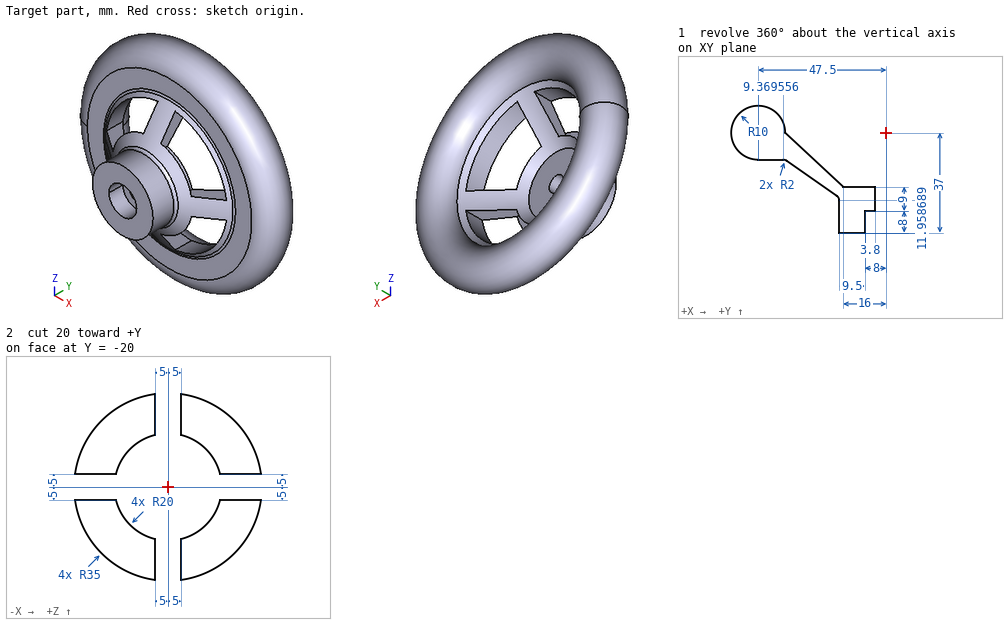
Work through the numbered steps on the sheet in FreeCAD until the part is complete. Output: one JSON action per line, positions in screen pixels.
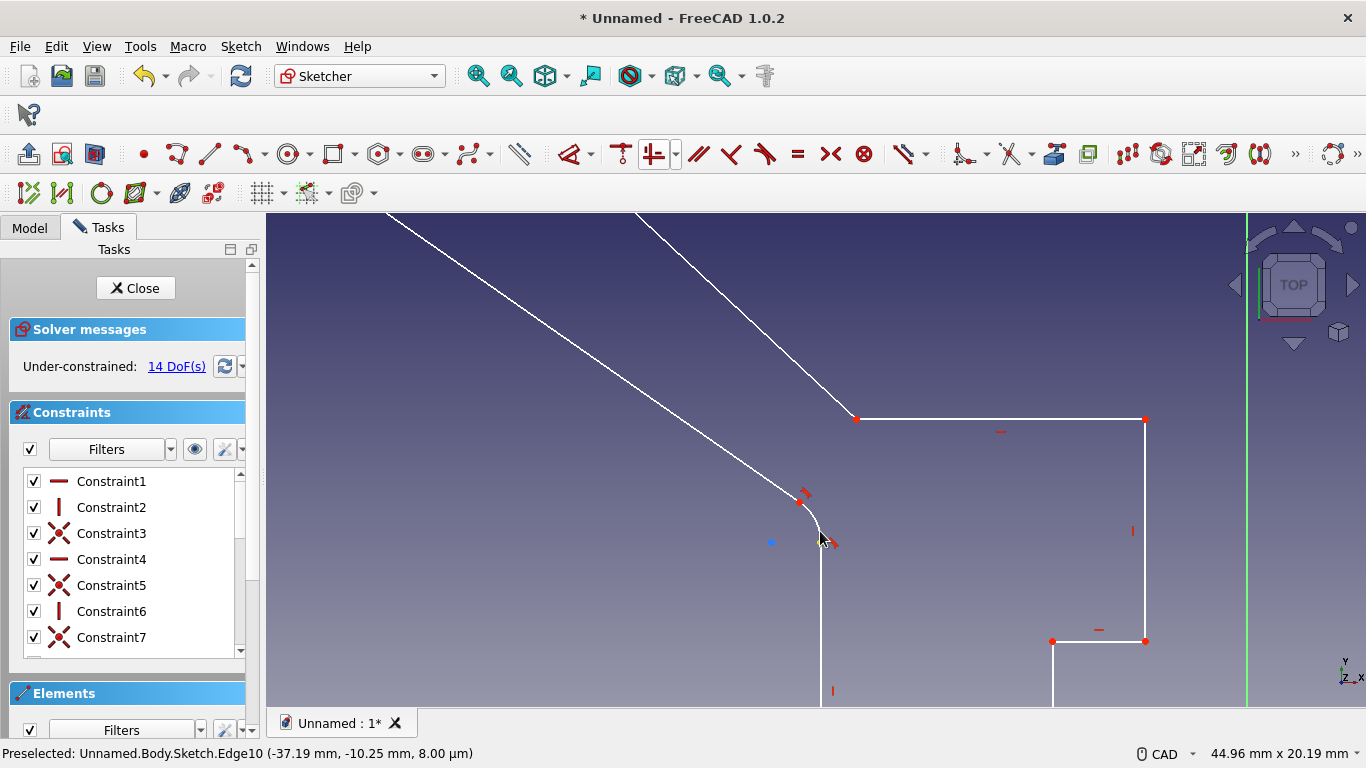
{"action": "left_click", "coordinate": [819, 529]}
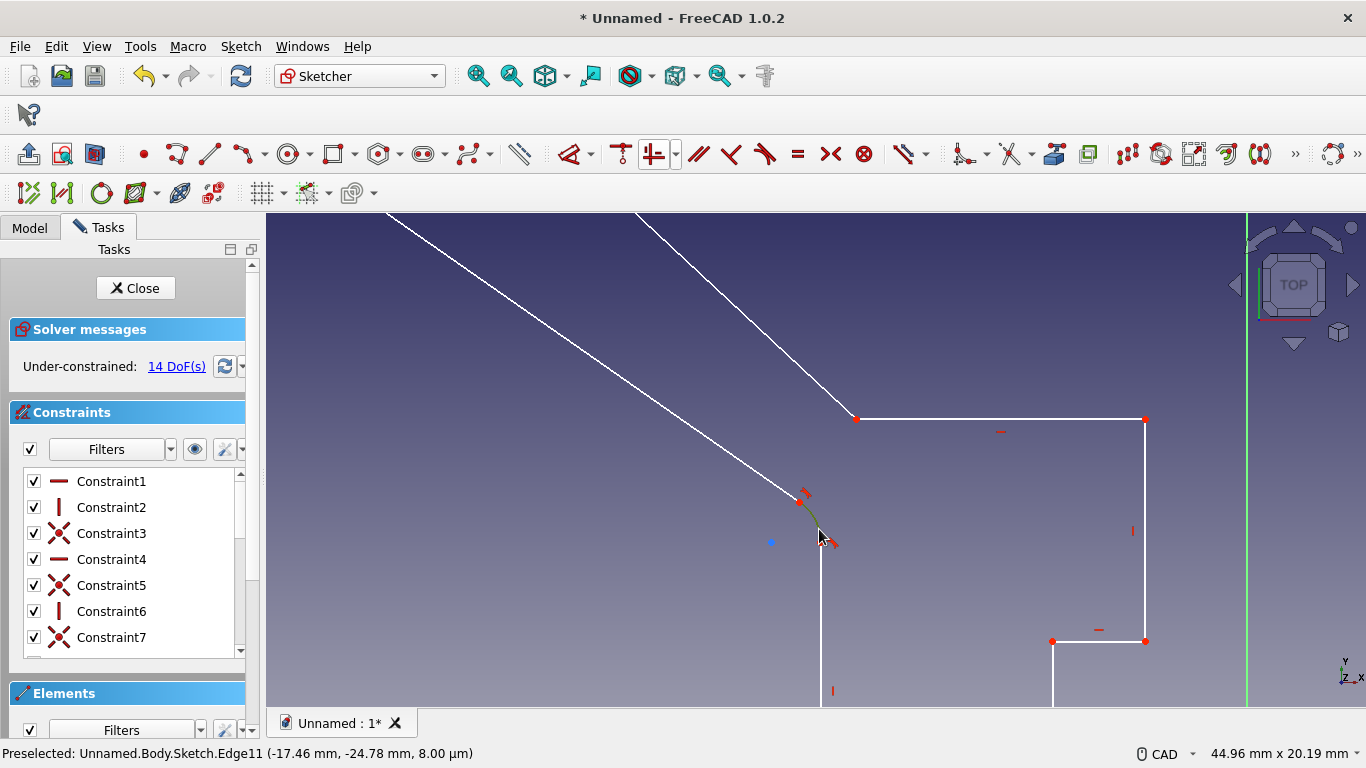
{"action": "key", "text": "e"}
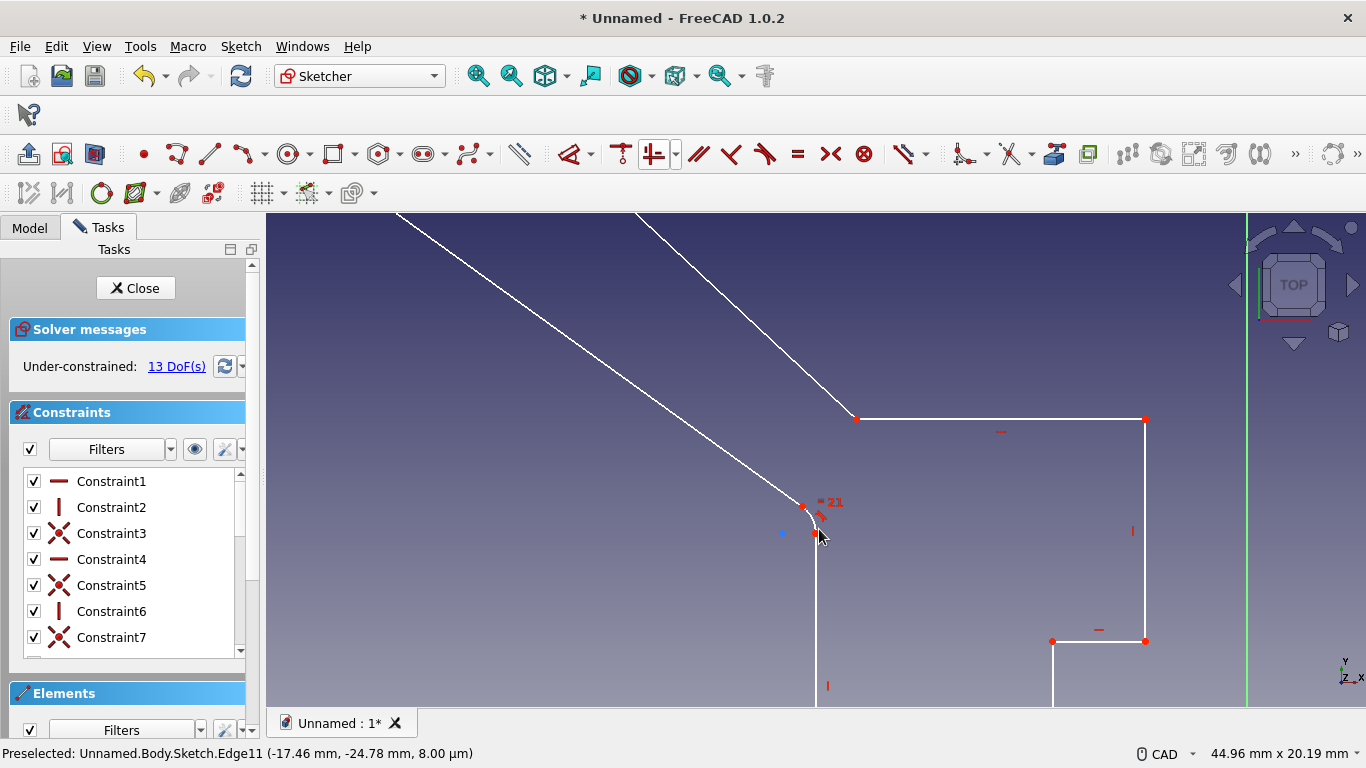
{"action": "scroll", "coordinate": [820, 531], "scroll_direction": "down", "scroll_amount": 6}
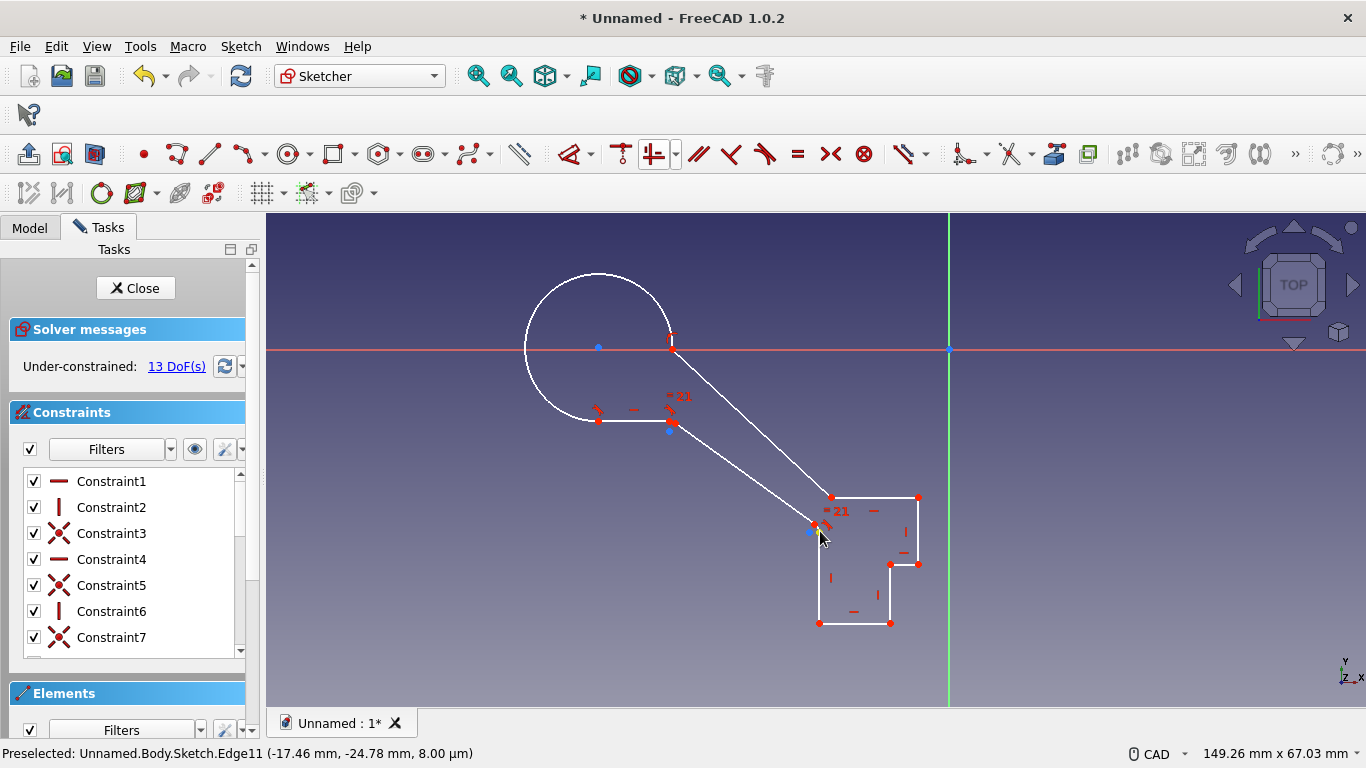
{"action": "left_click", "coordinate": [599, 348]}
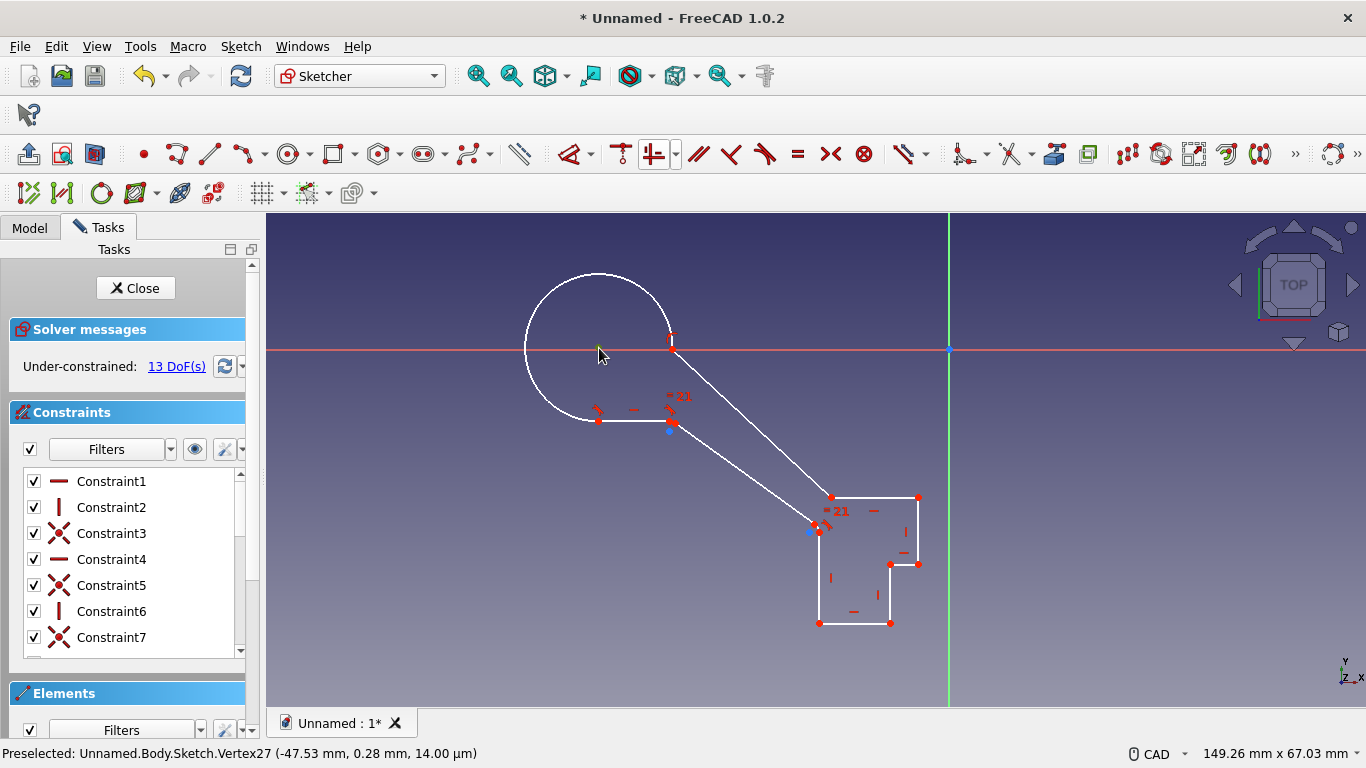
{"action": "left_click", "coordinate": [359, 350]}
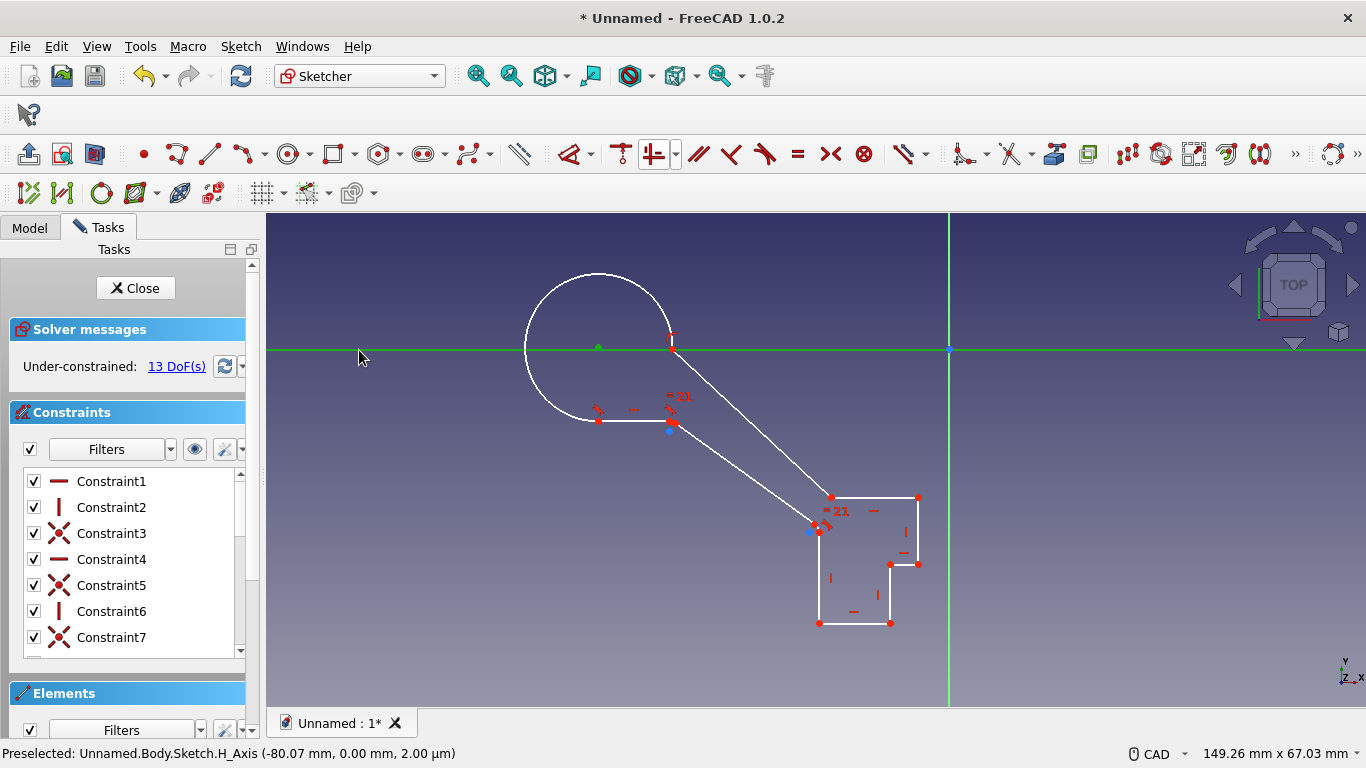
{"action": "key", "text": "c"}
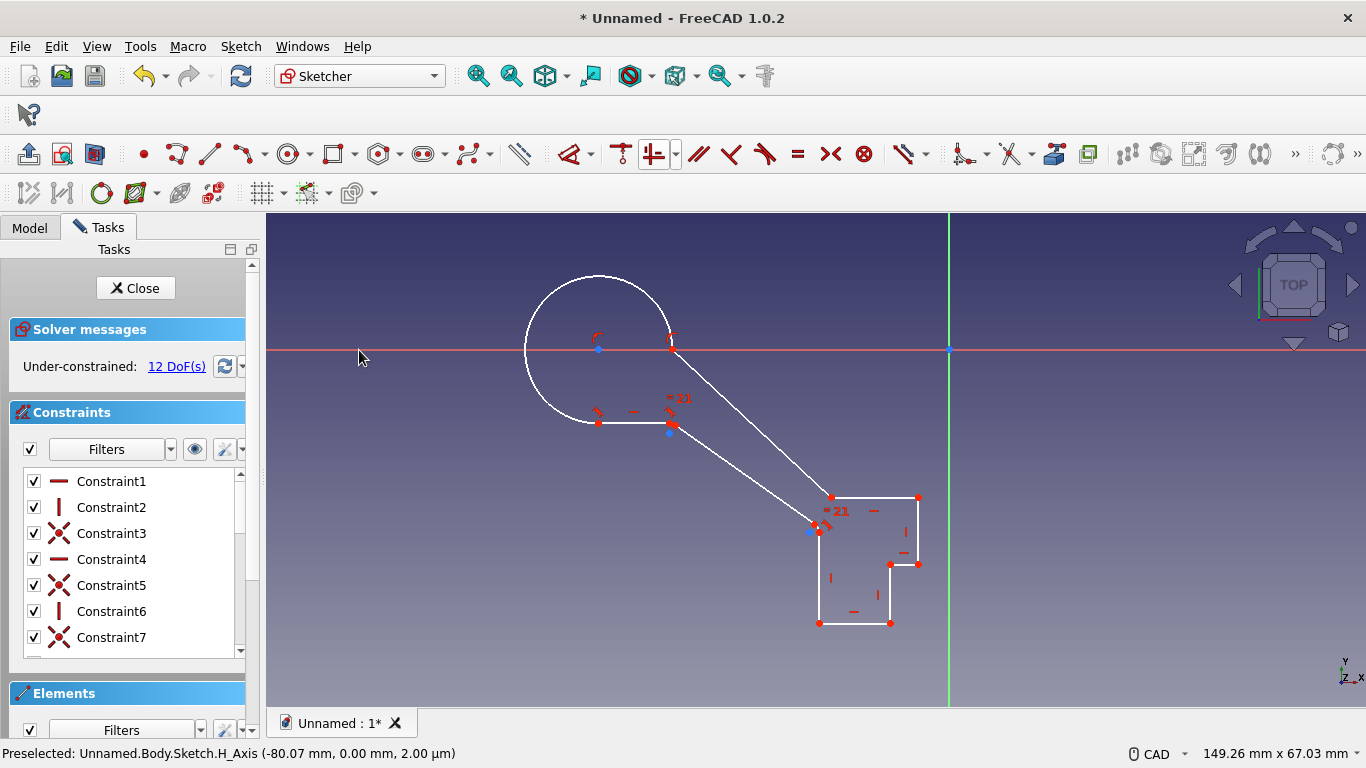
{"action": "key", "text": "d"}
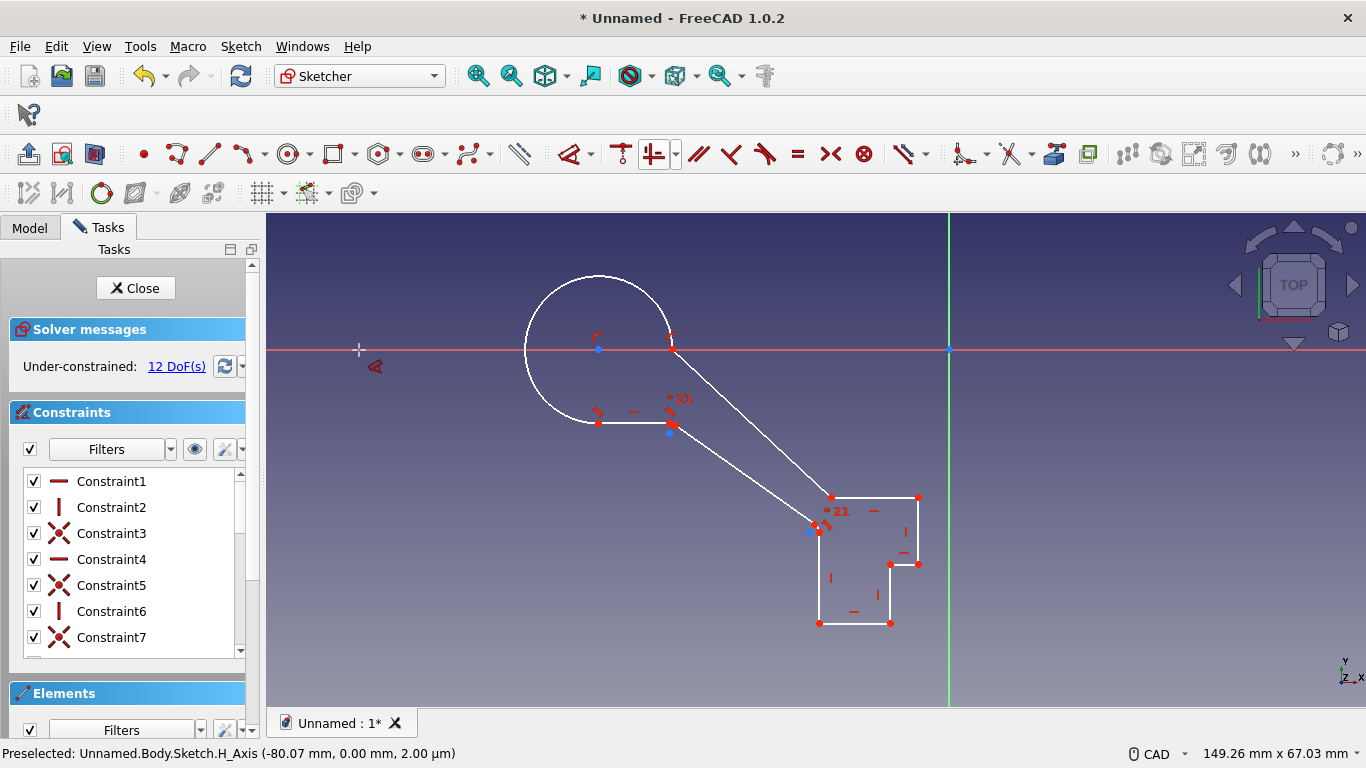
{"action": "scroll", "coordinate": [673, 424], "scroll_direction": "up", "scroll_amount": 8}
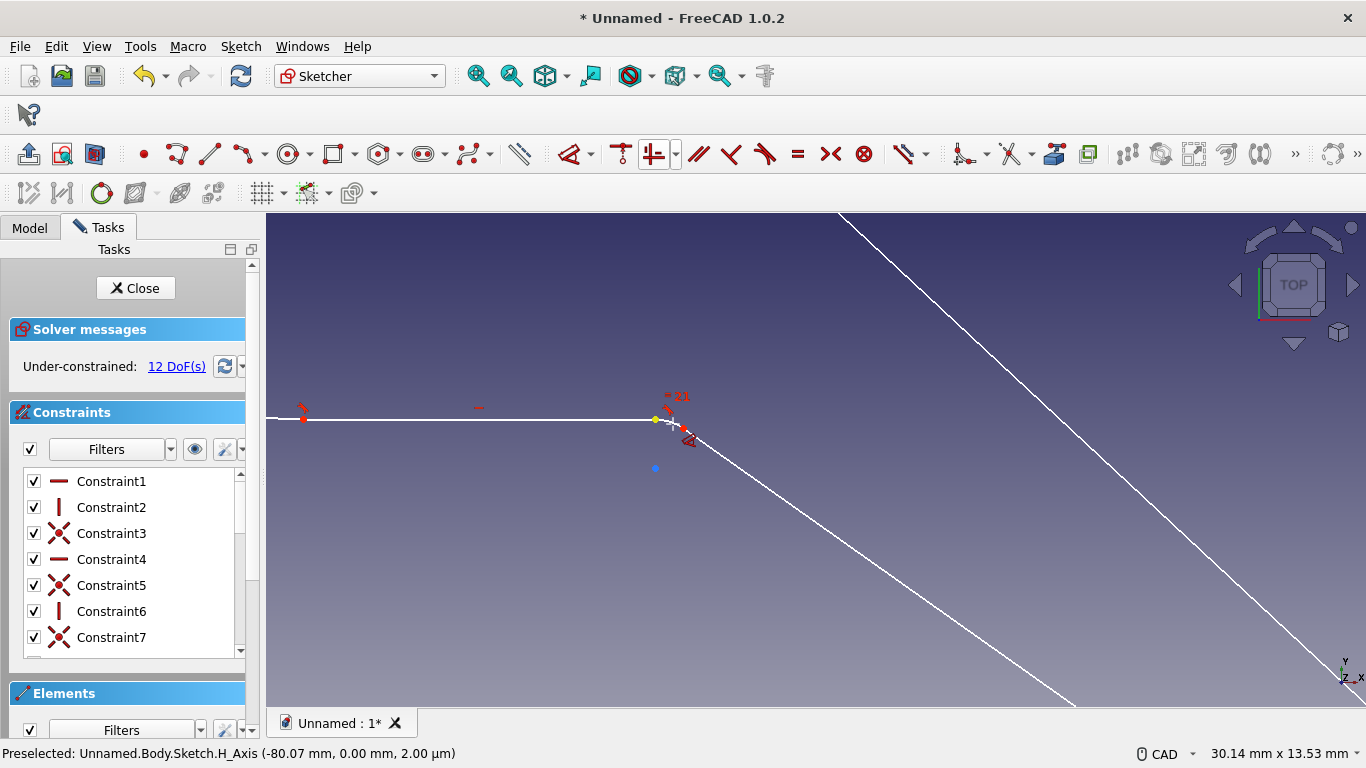
{"action": "left_click", "coordinate": [670, 422]}
{"action": "left_click", "coordinate": [680, 391]}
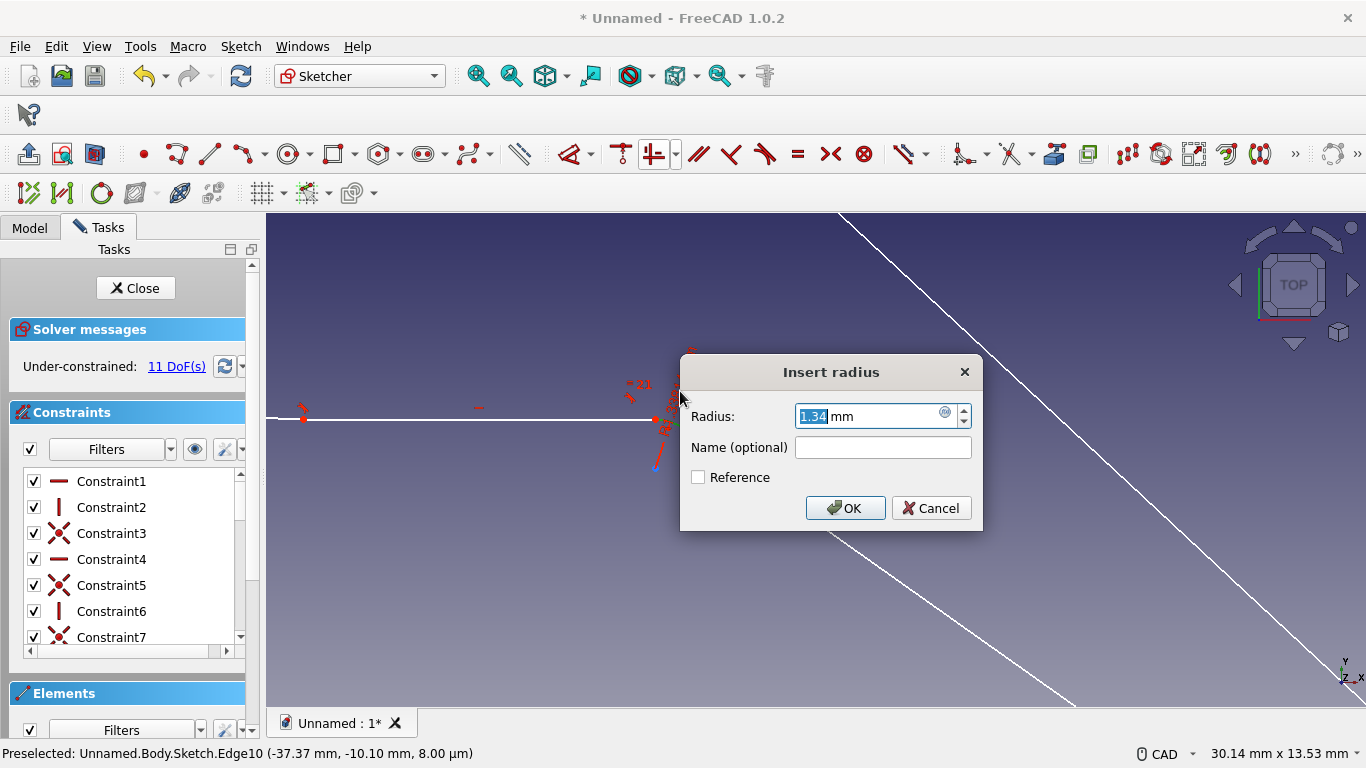
{"action": "type", "text": "2"}
{"action": "key", "text": "Return"}